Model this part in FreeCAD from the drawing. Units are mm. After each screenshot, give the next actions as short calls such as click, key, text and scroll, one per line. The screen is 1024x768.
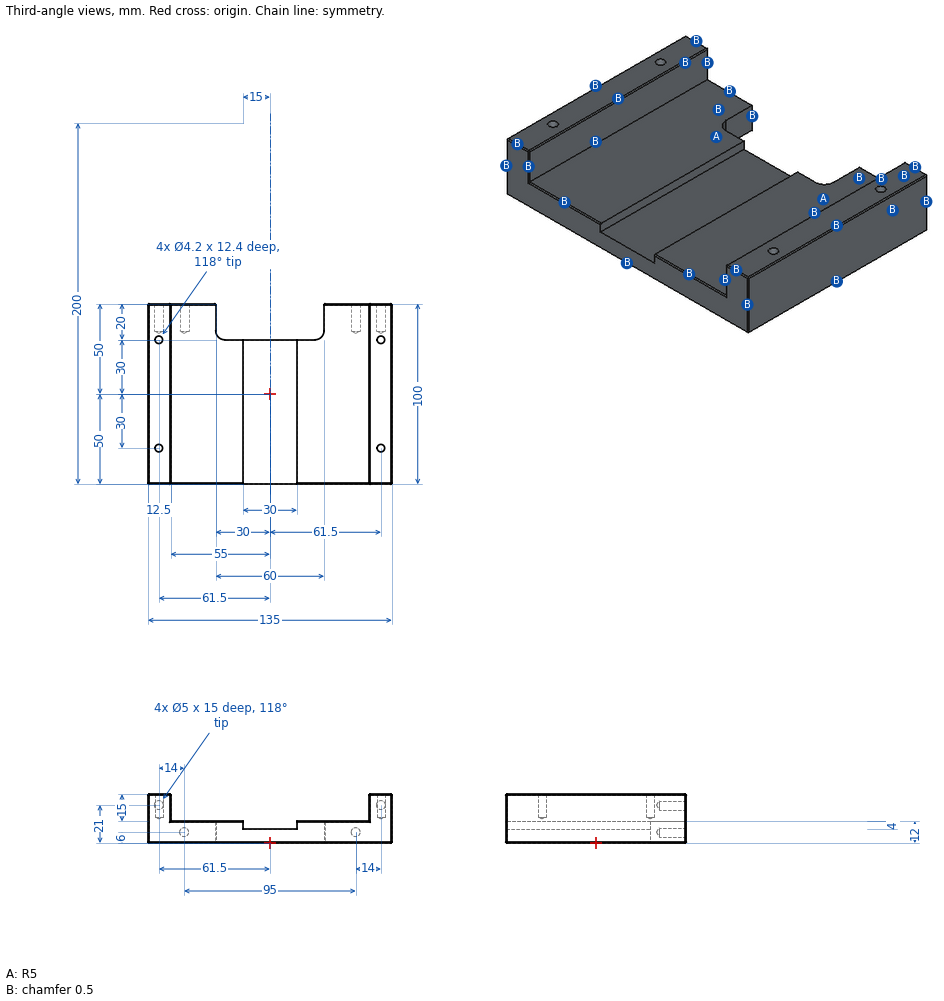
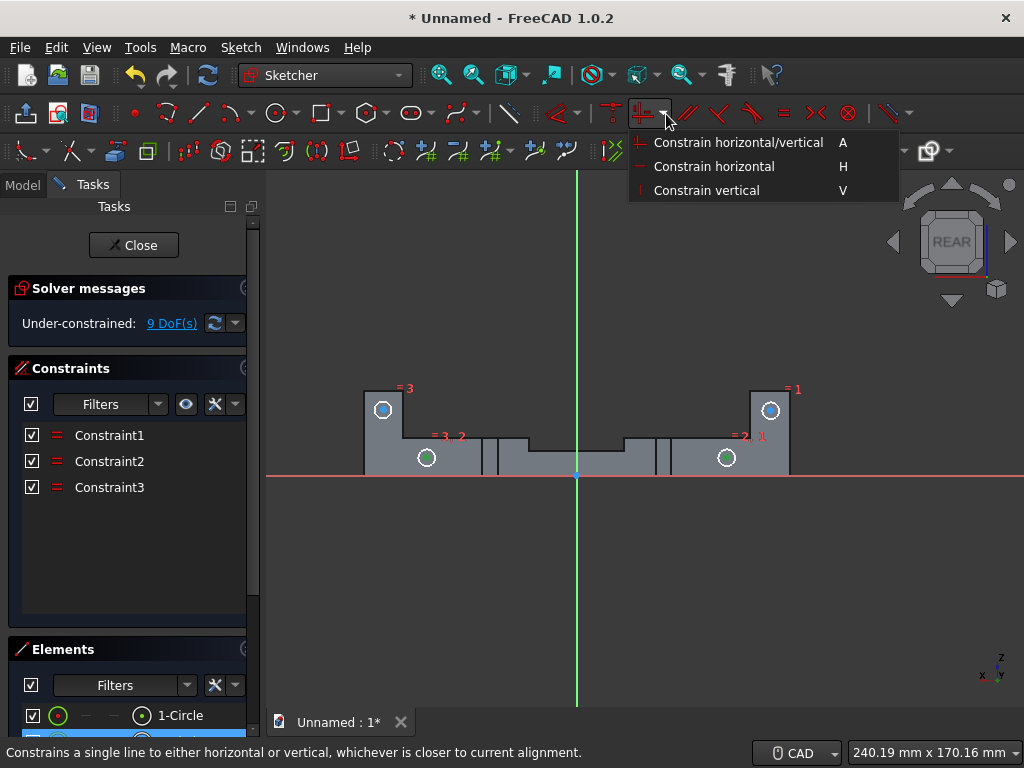
click(764, 166)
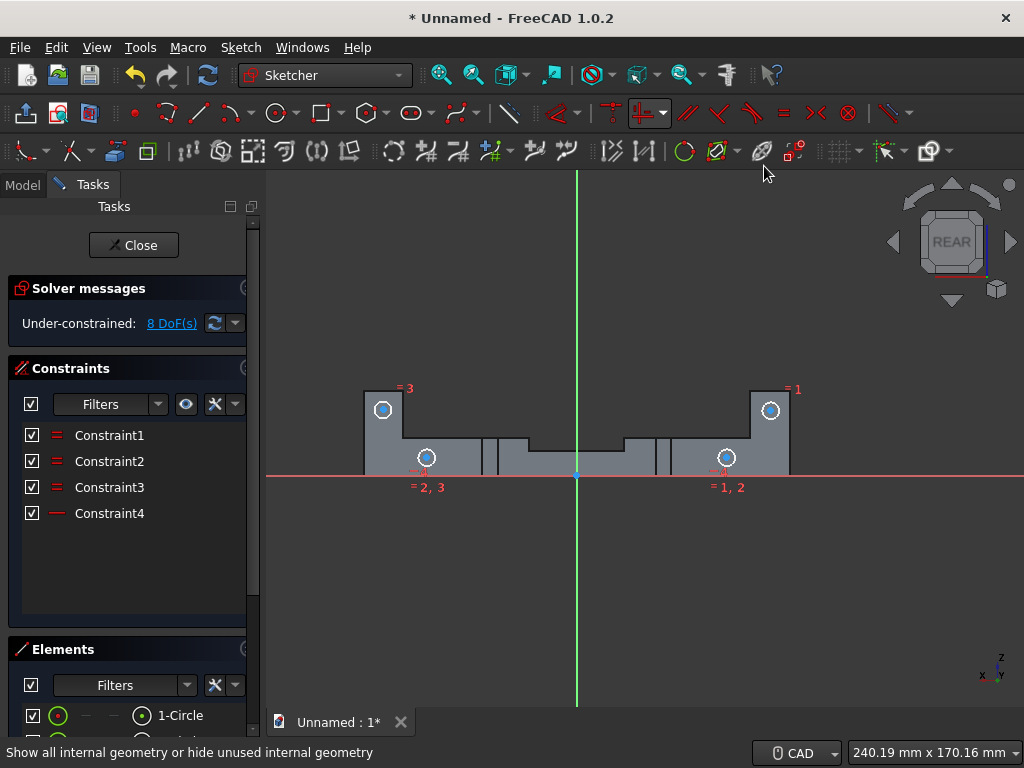
click(771, 411)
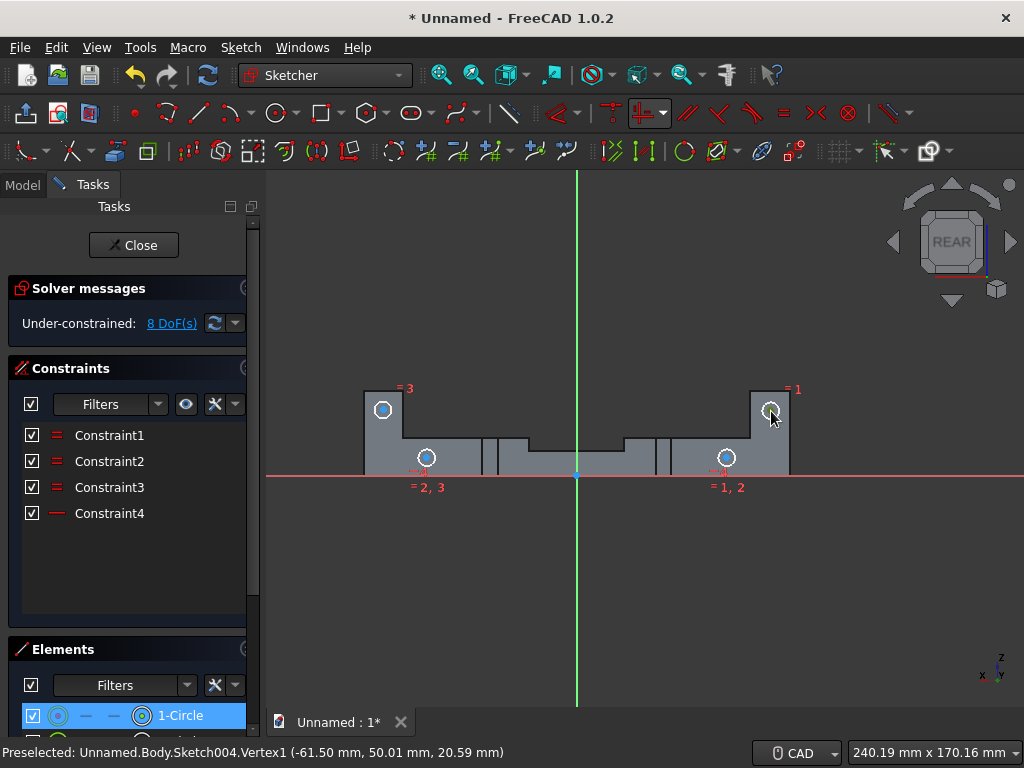
click(383, 410)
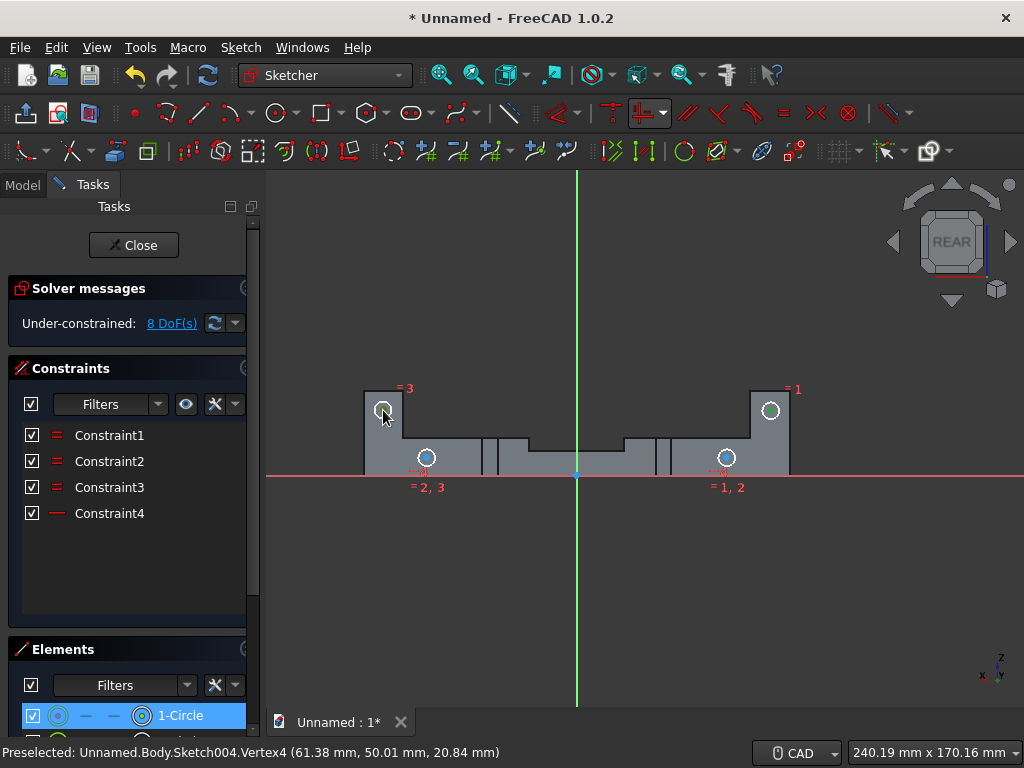
click(666, 114)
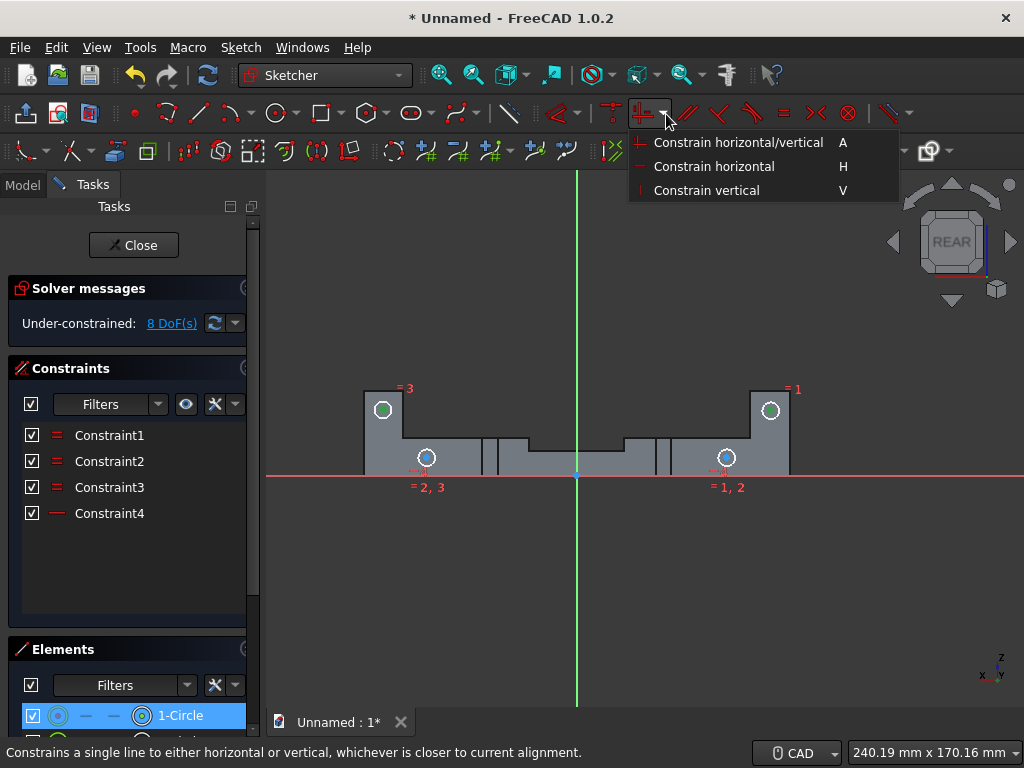
click(764, 166)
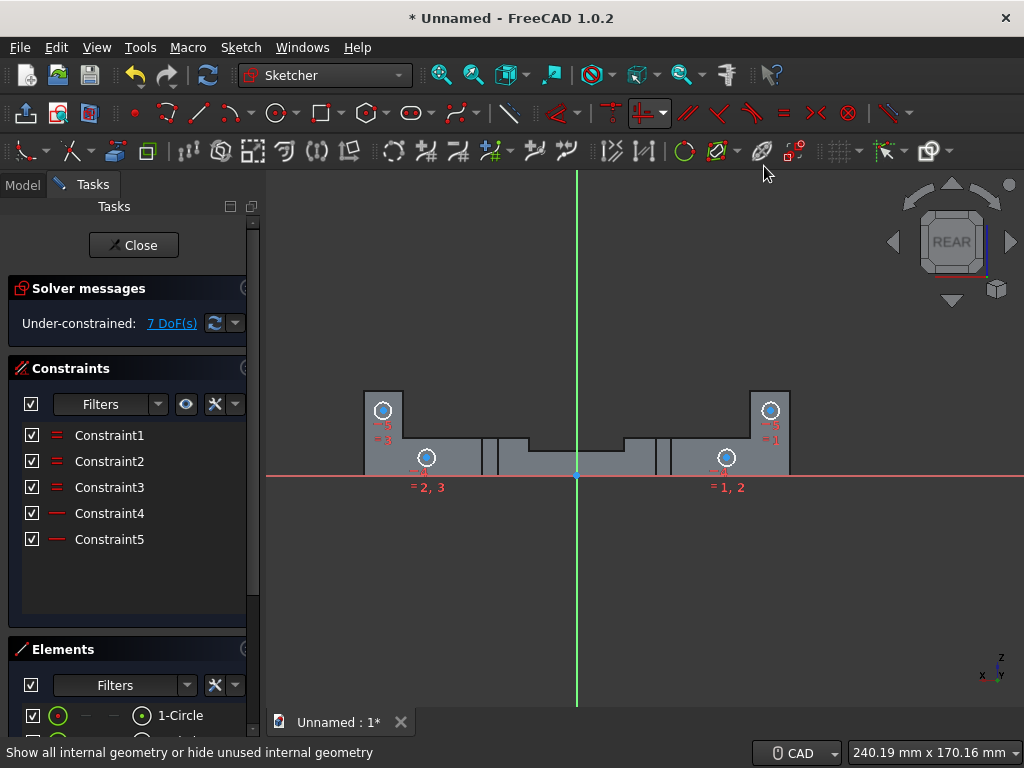
key(d)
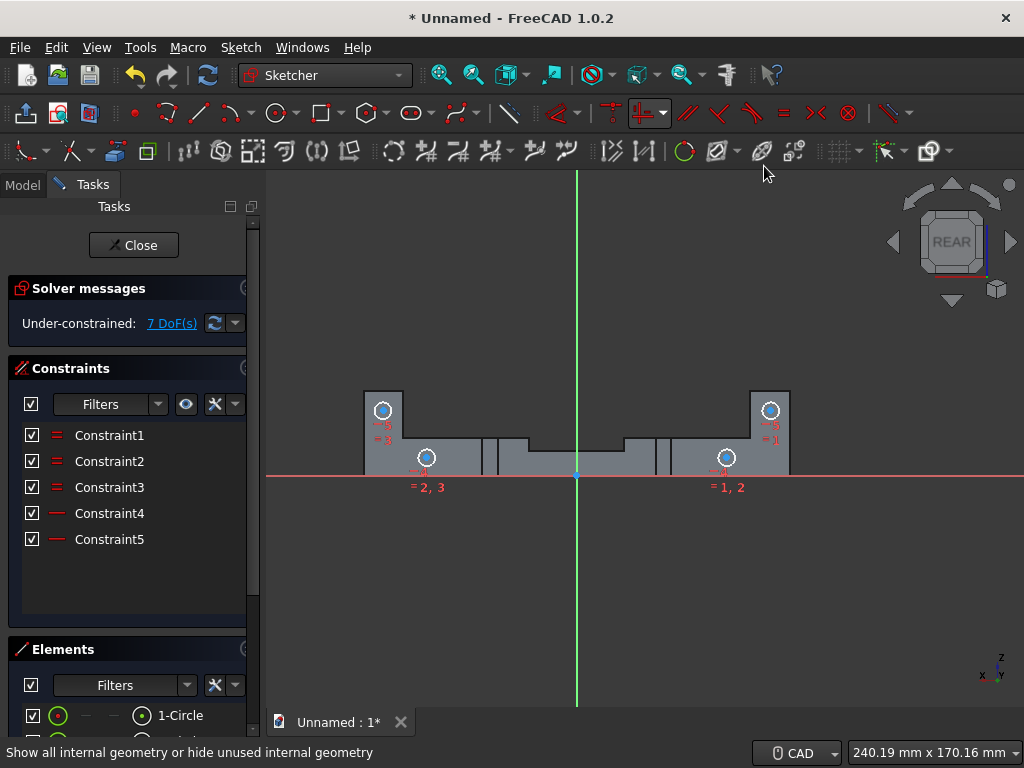
scroll(771, 402, up, 5)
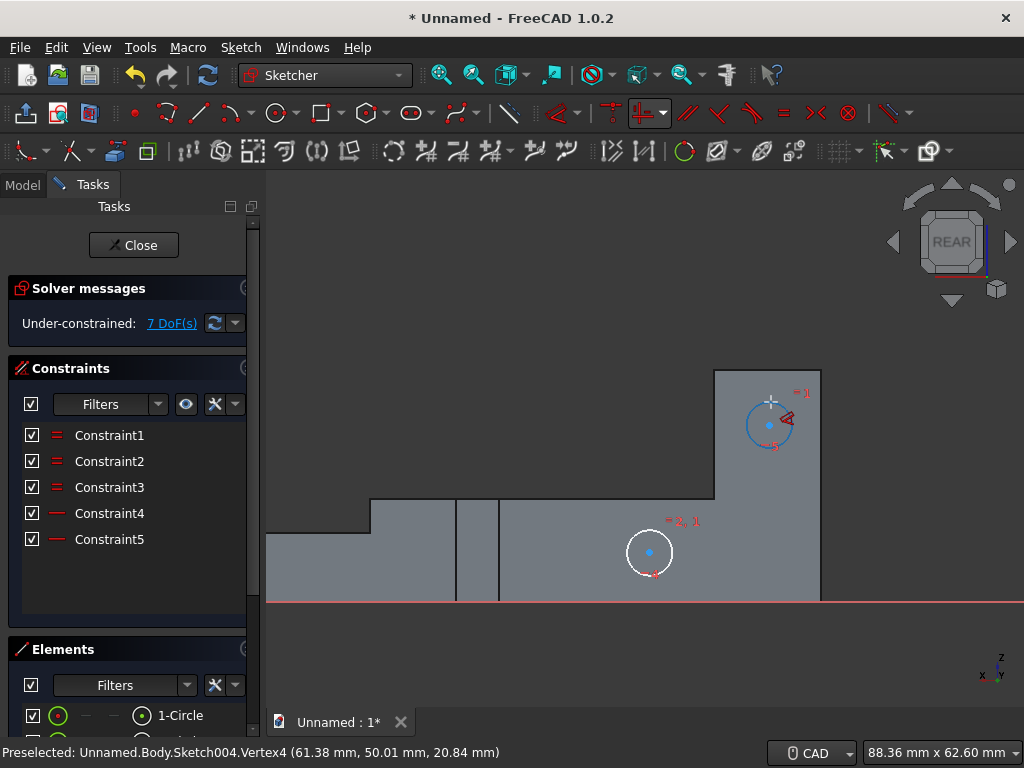
click(770, 402)
click(771, 370)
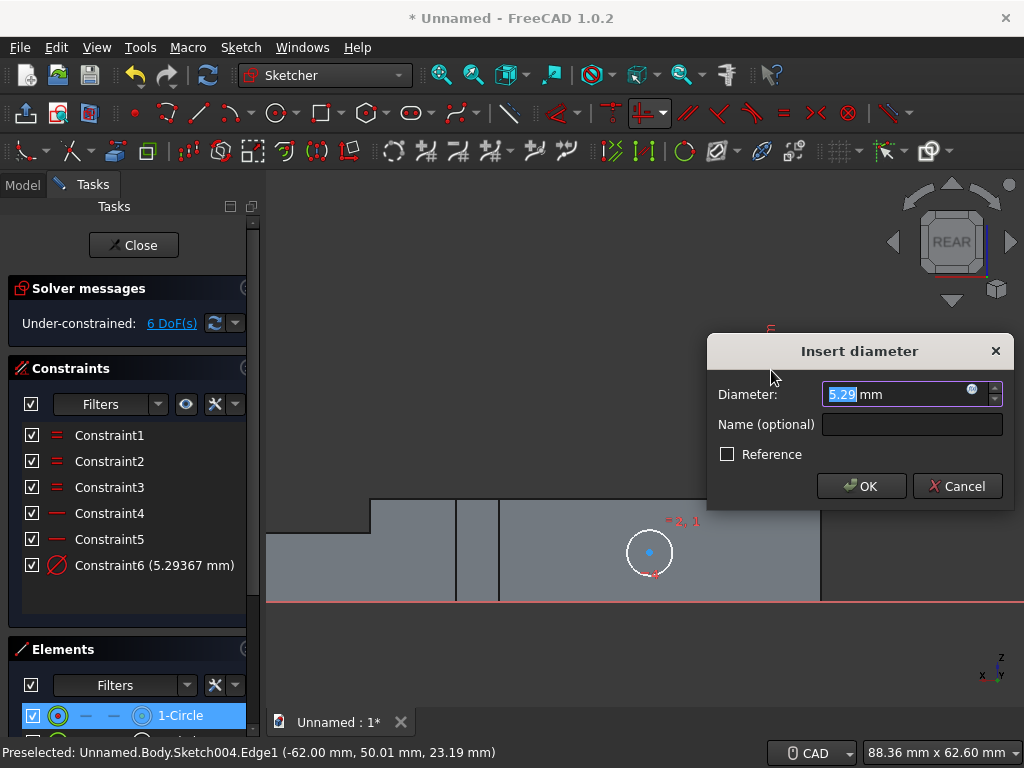
text(5)
key(Return)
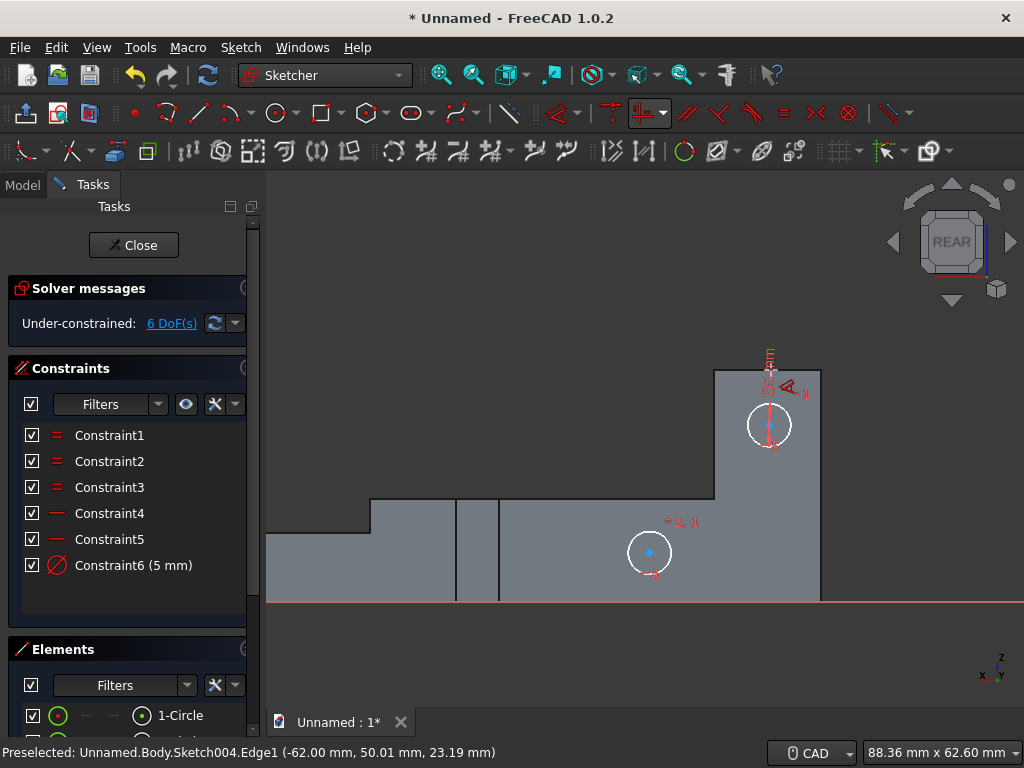
click(650, 553)
click(684, 577)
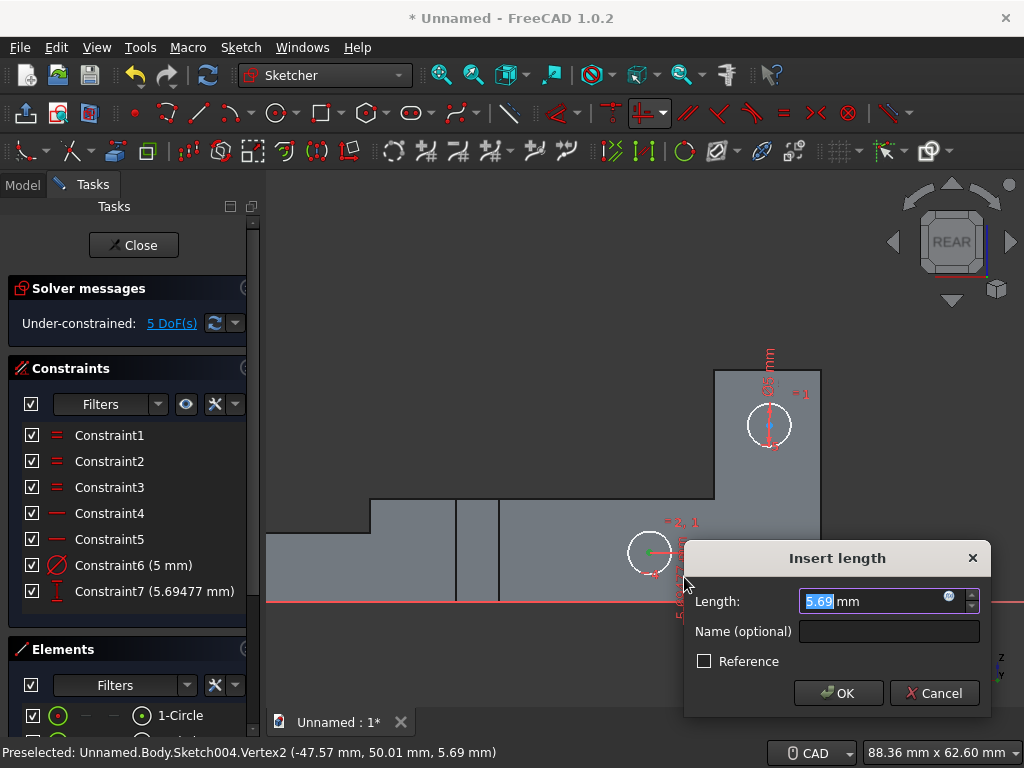
text(6)
key(Return)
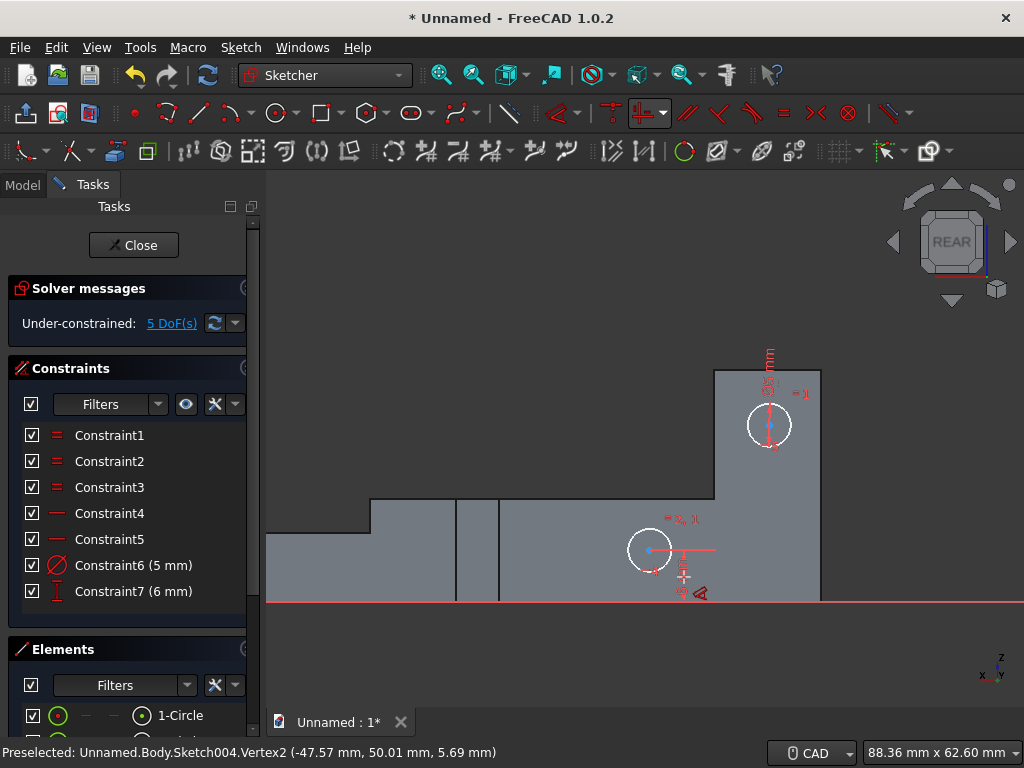
click(769, 425)
click(803, 513)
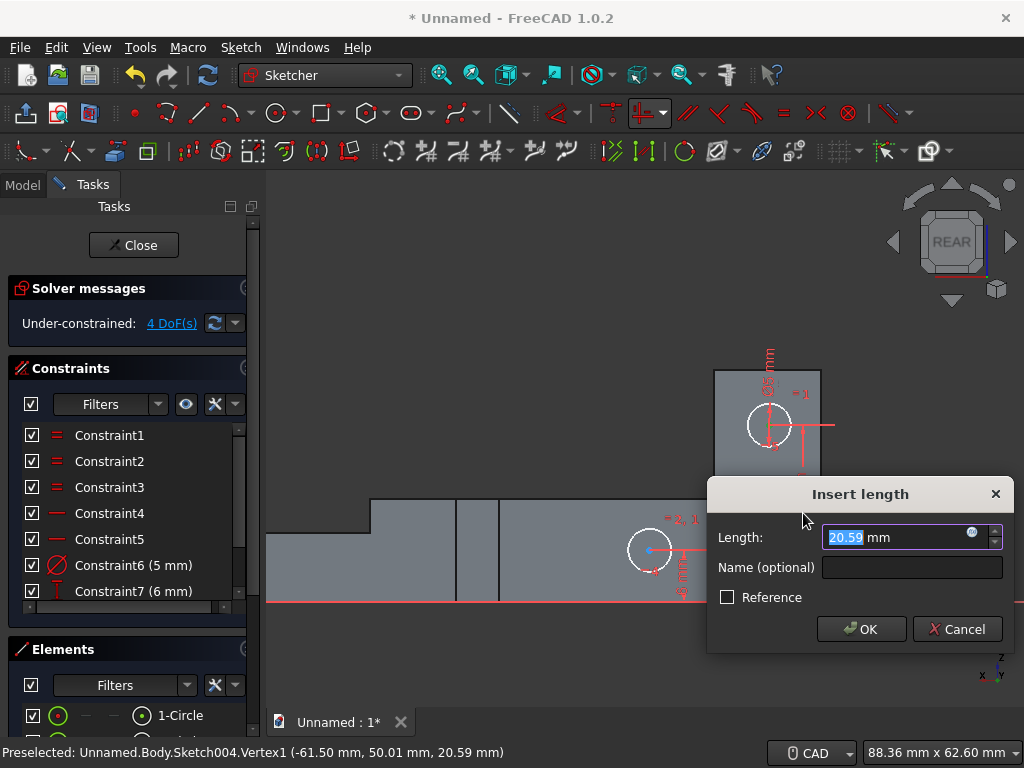
text(21)
key(Return)